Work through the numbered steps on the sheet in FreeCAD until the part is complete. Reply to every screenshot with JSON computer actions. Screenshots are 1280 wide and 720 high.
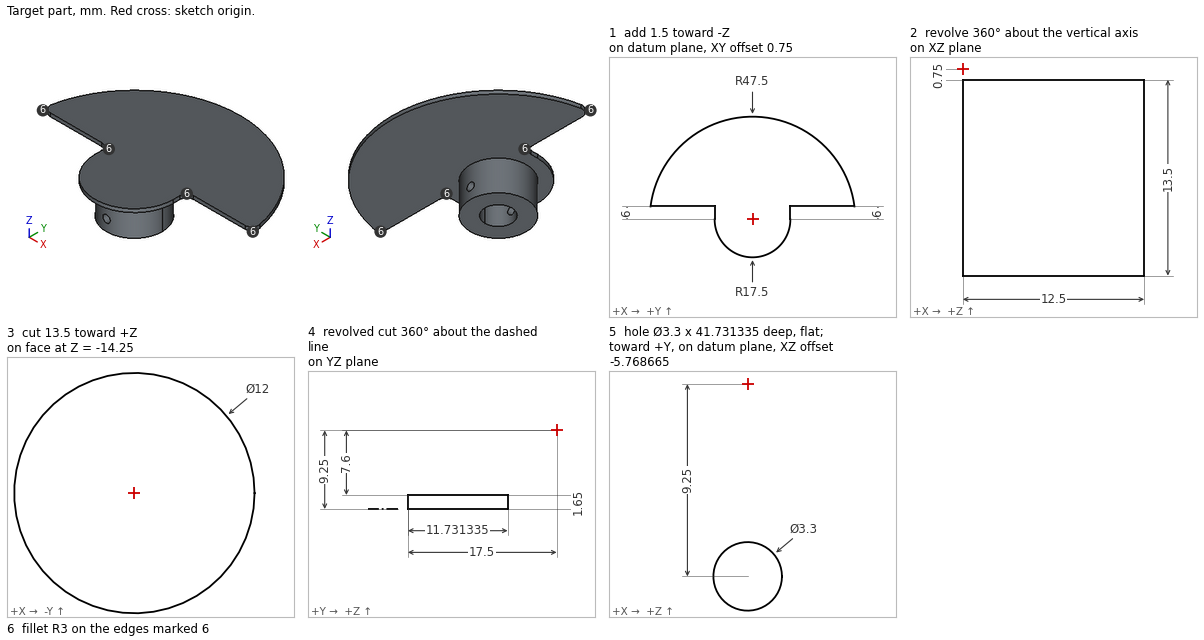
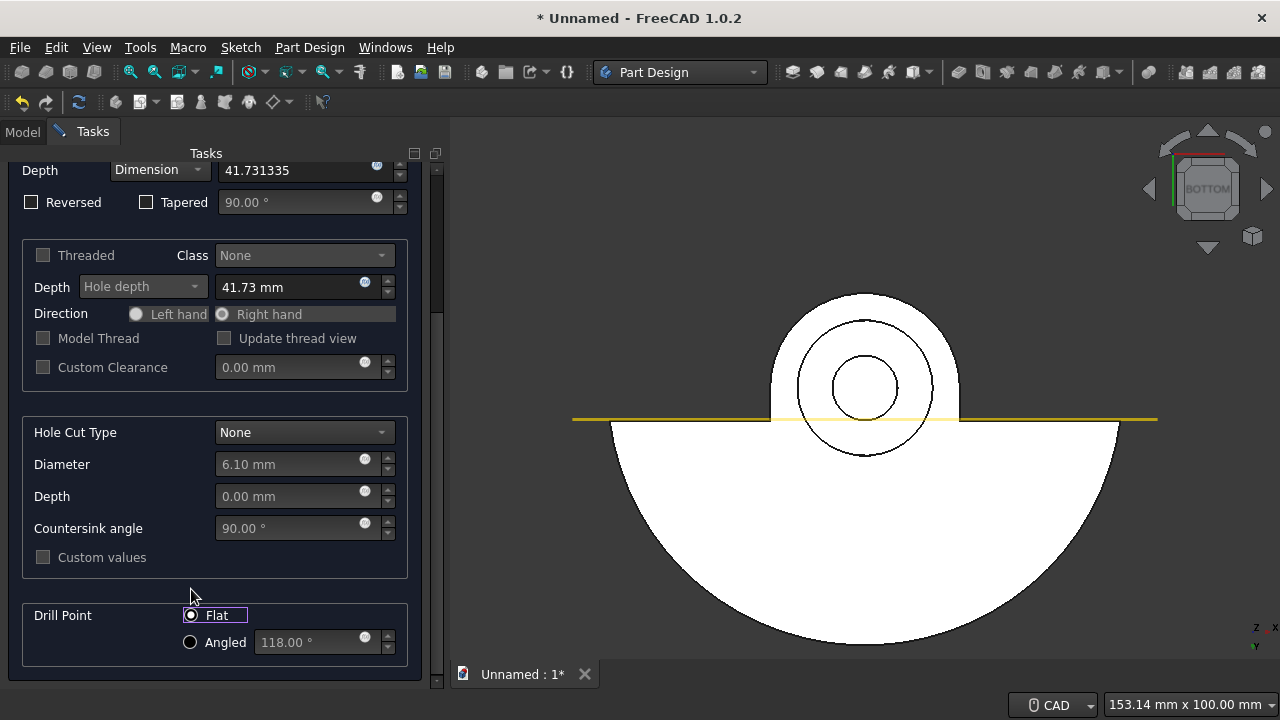
{"action": "scroll", "coordinate": [437, 426], "scroll_direction": "up", "scroll_amount": 5}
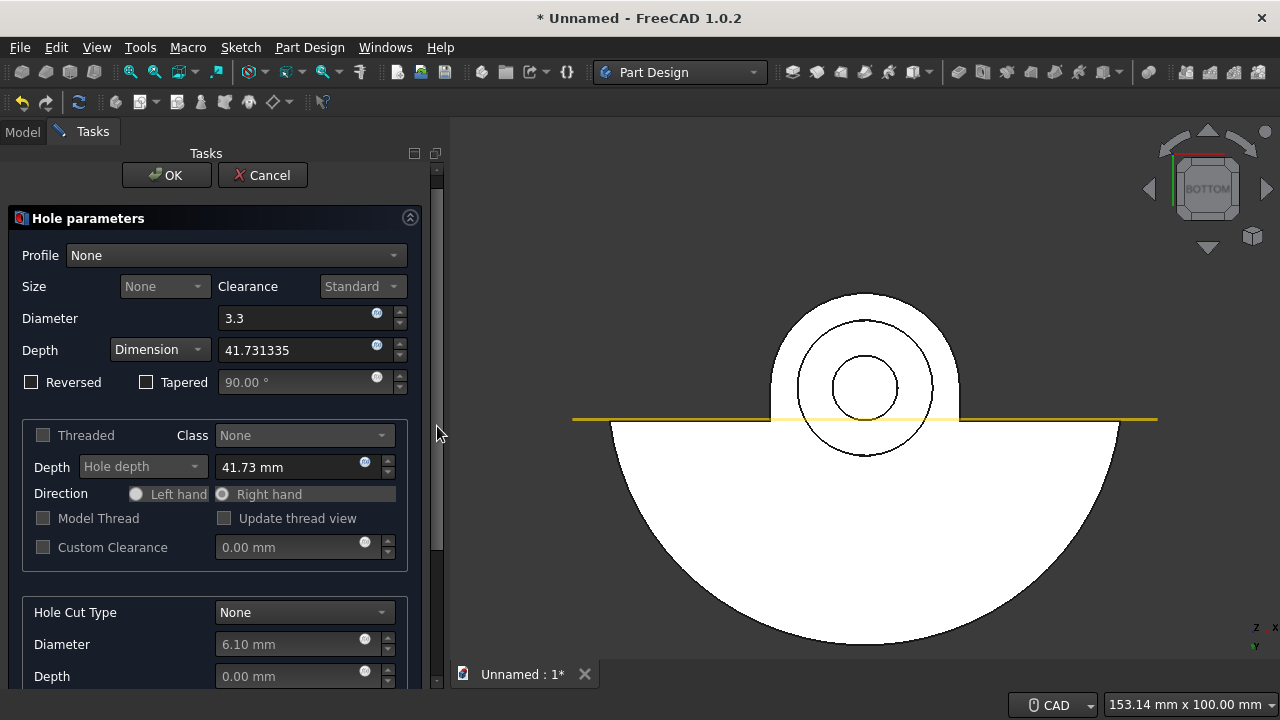
{"action": "left_click", "coordinate": [167, 192]}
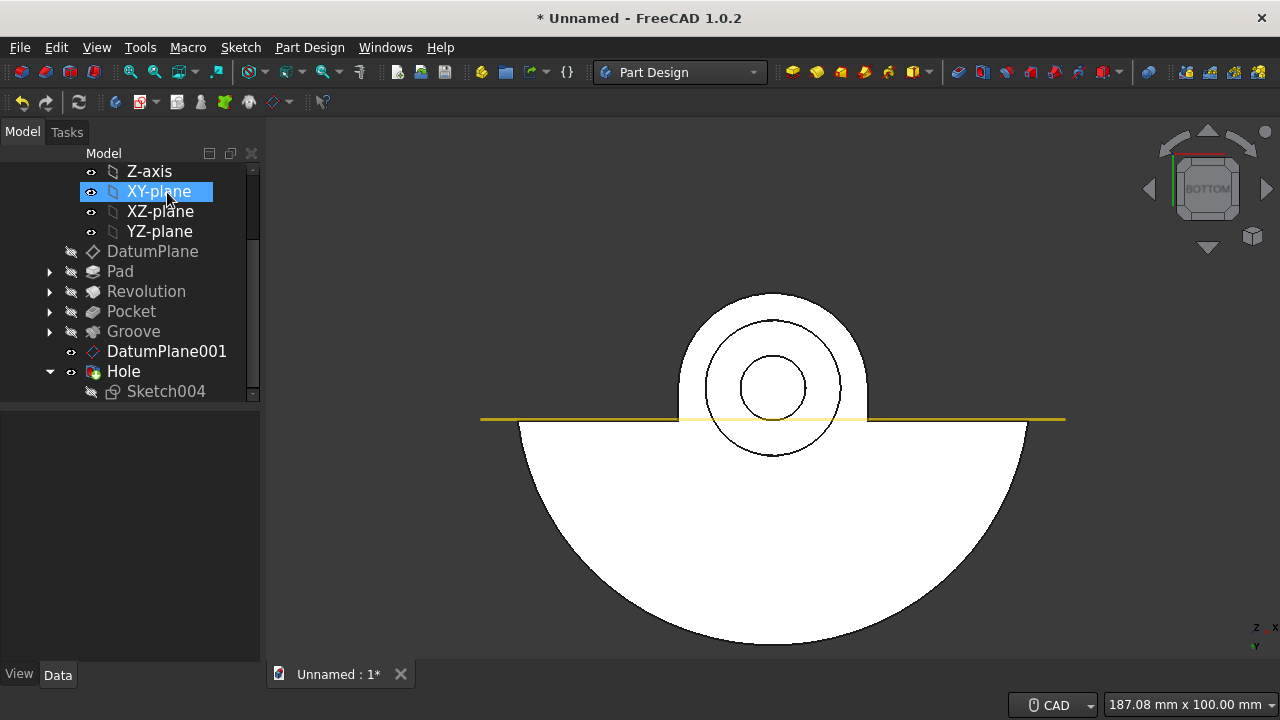
{"action": "left_click", "coordinate": [116, 352]}
{"action": "key", "text": "space"}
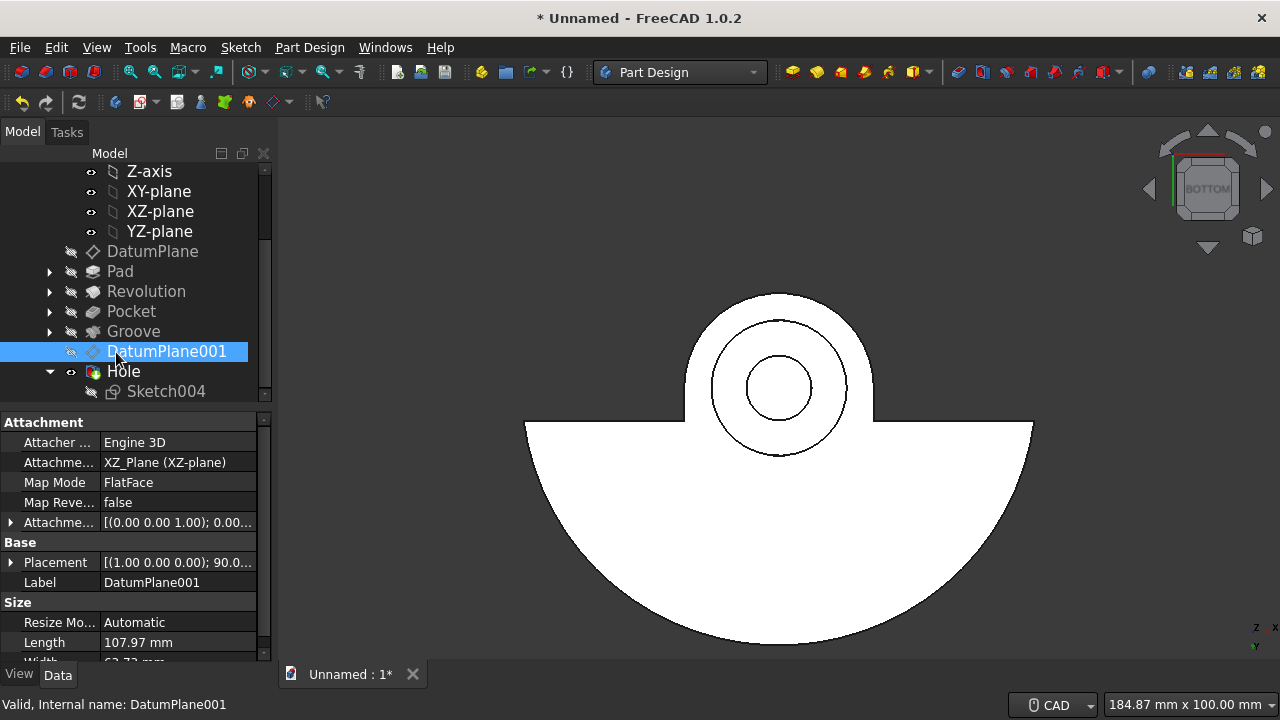
{"action": "scroll", "coordinate": [684, 420], "scroll_direction": "up", "scroll_amount": 8}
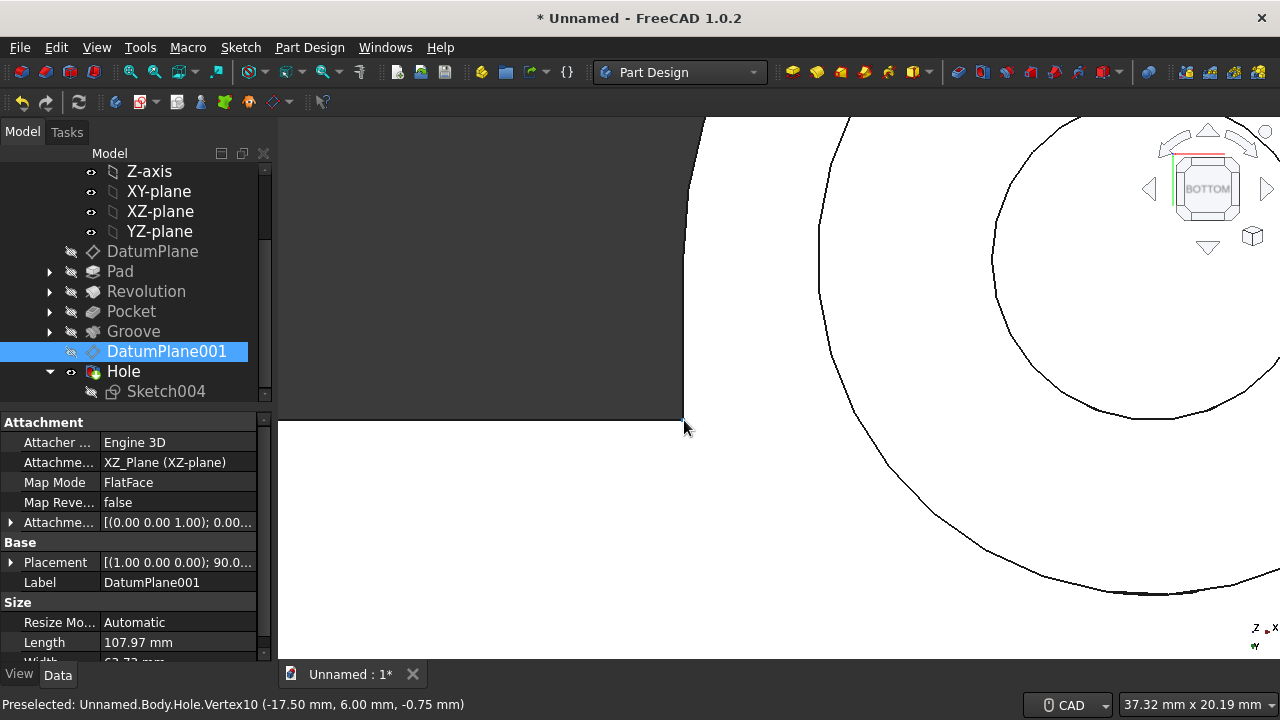
{"action": "key", "text": "v f"}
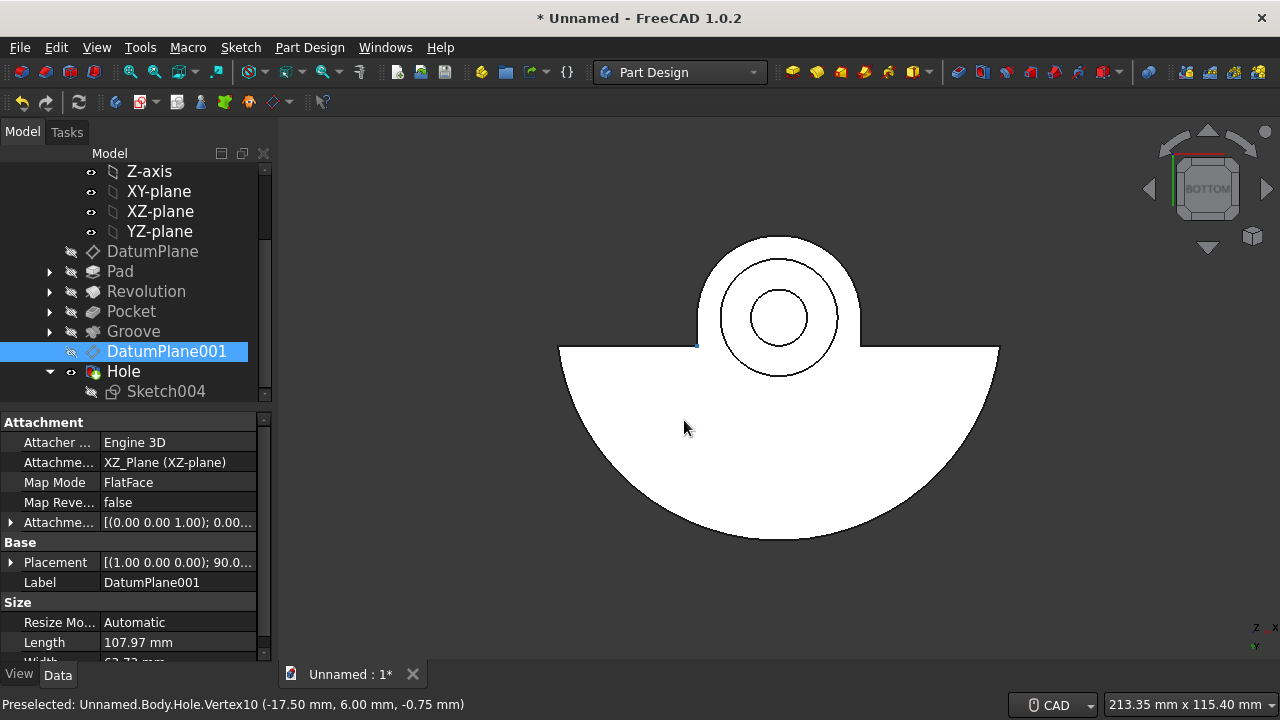
{"action": "key", "text": "0"}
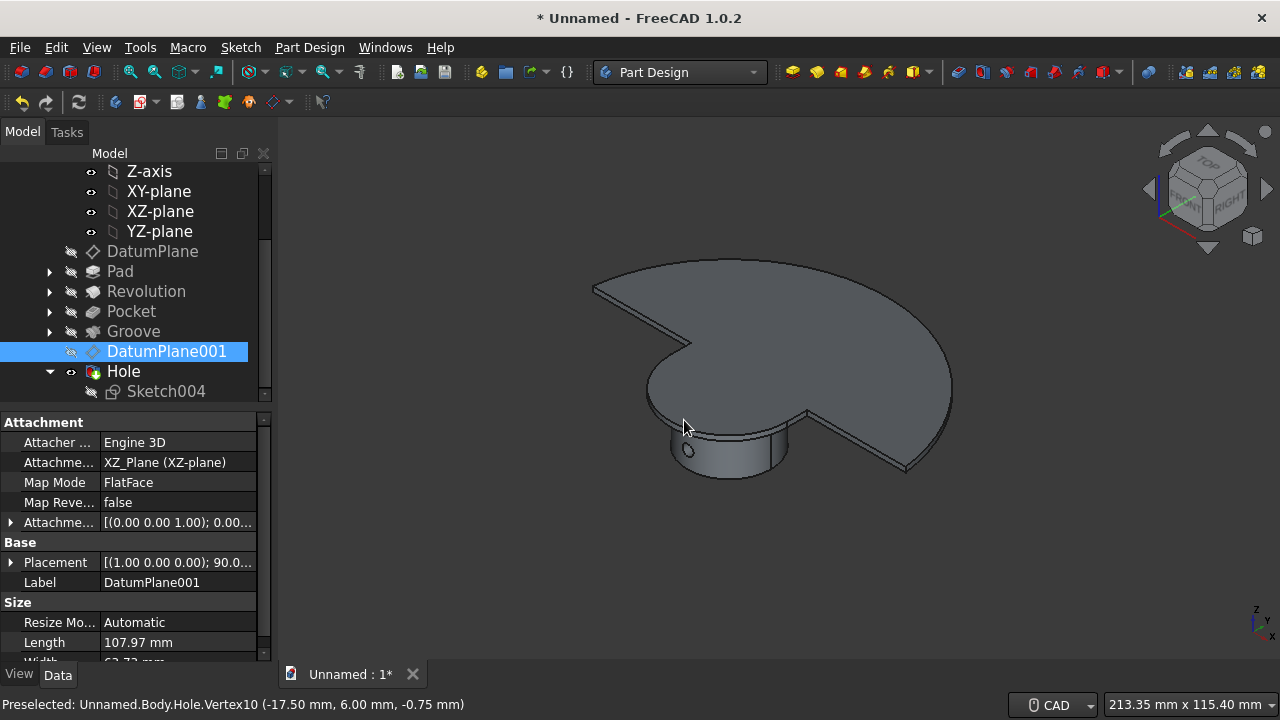
{"action": "scroll", "coordinate": [691, 345], "scroll_direction": "up", "scroll_amount": 9}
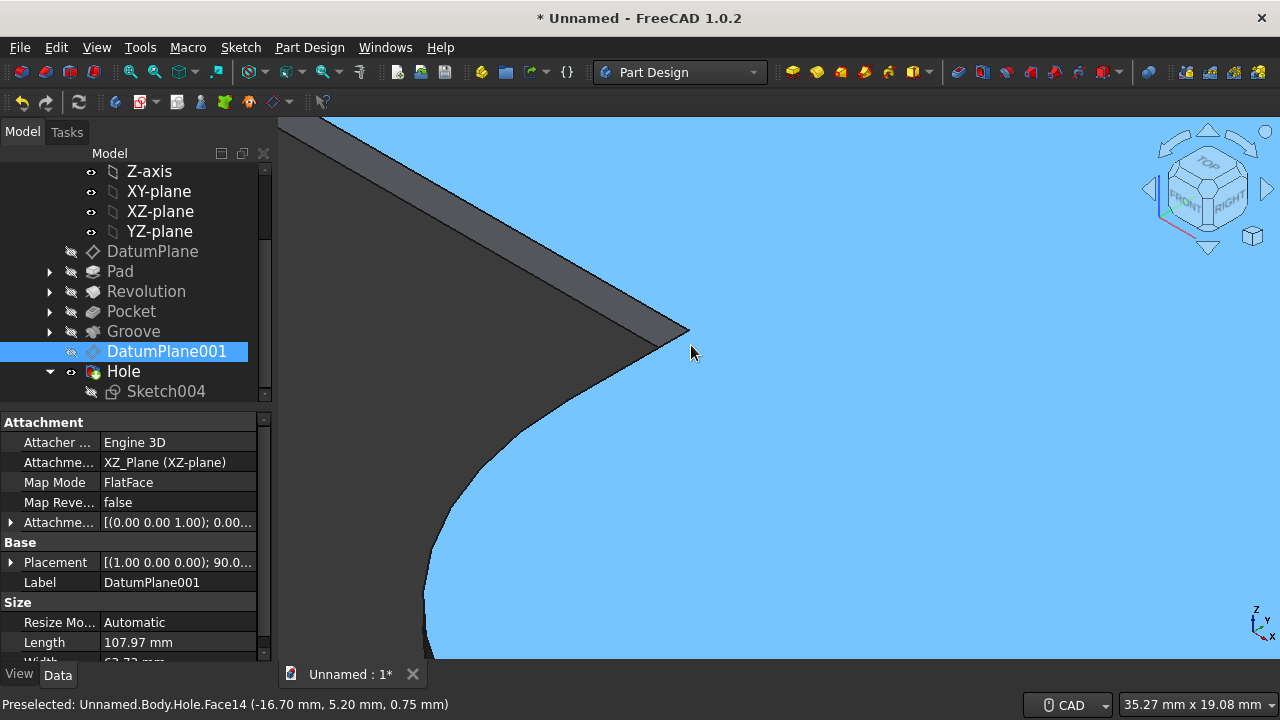
{"action": "left_click", "coordinate": [132, 72]}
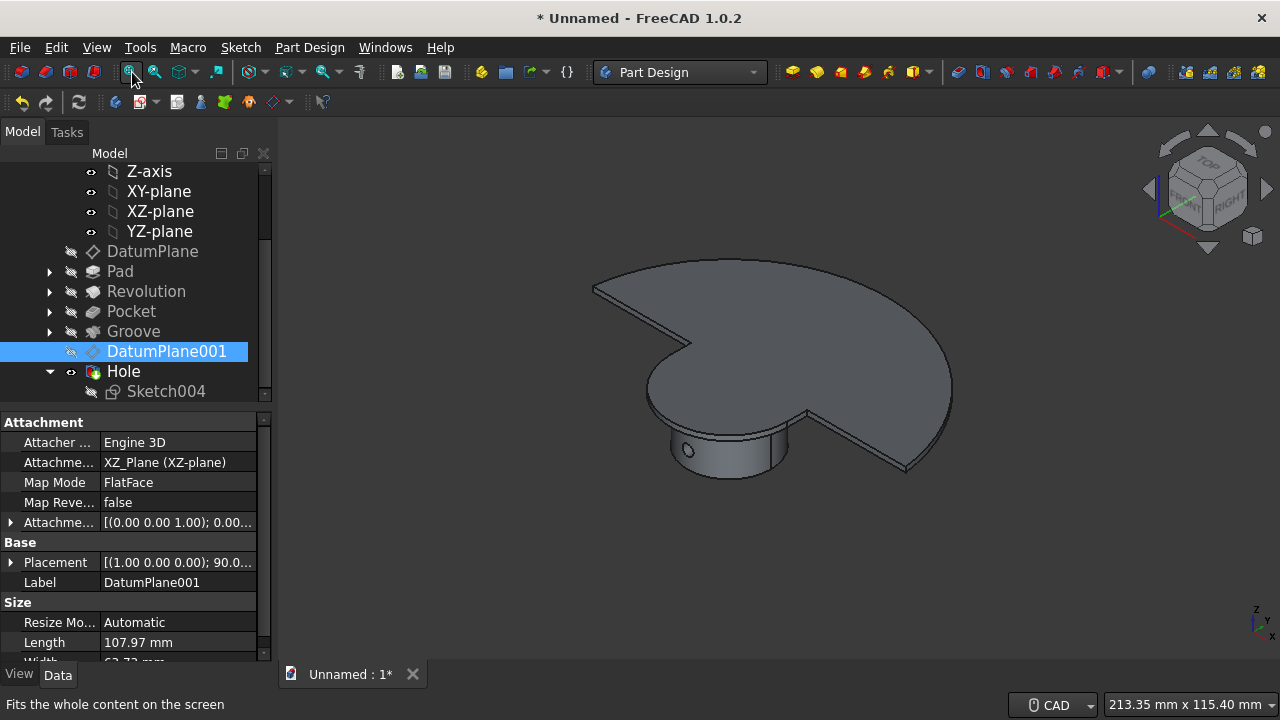
{"action": "key", "text": "2"}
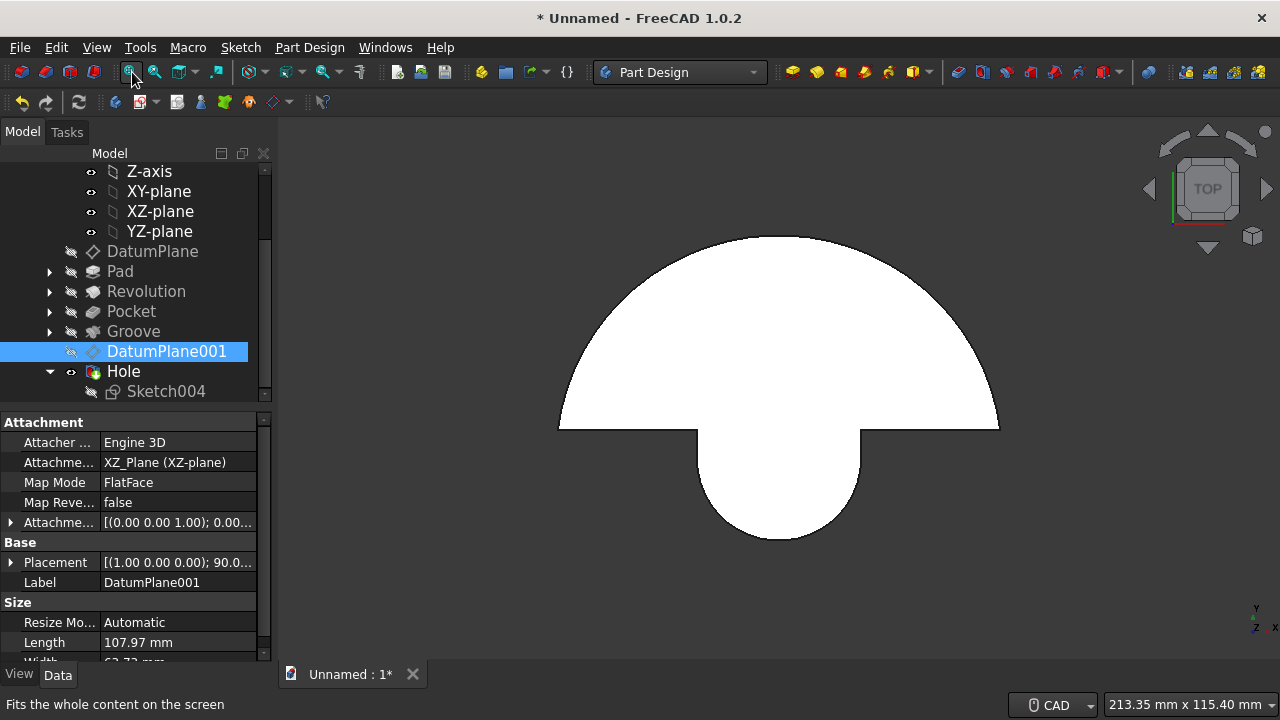
{"action": "scroll", "coordinate": [697, 429], "scroll_direction": "up", "scroll_amount": 9}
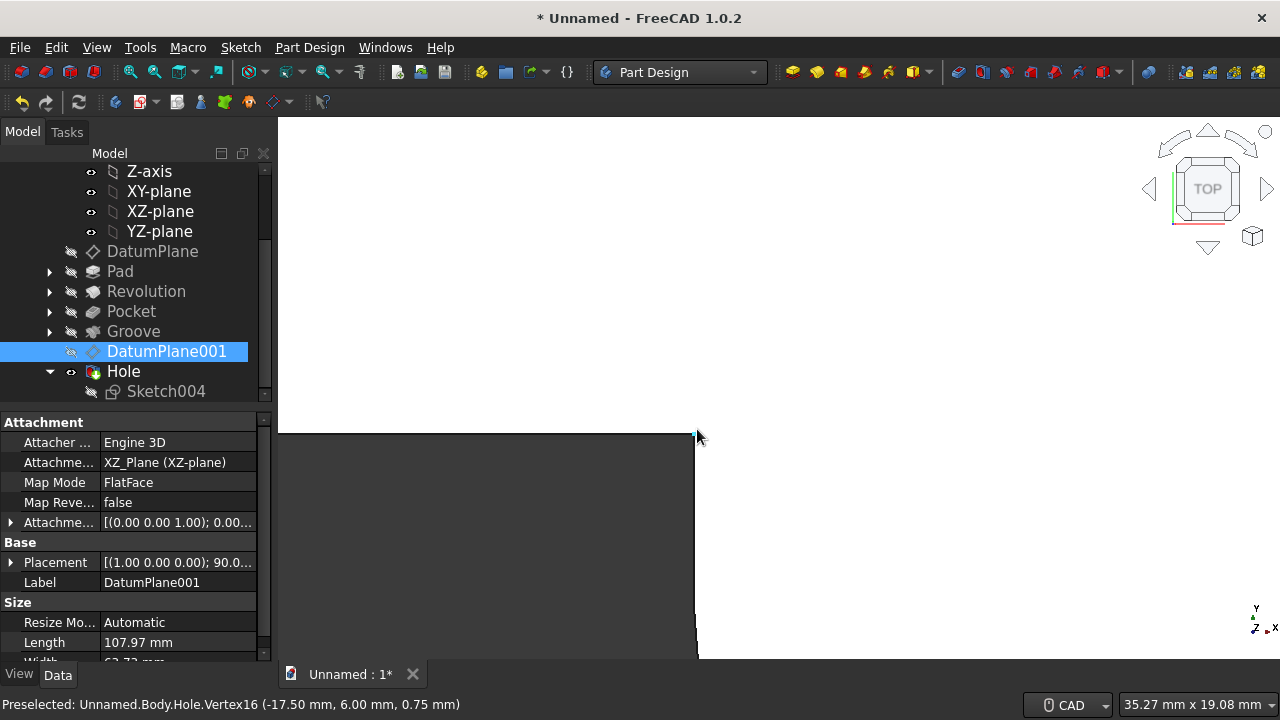
{"action": "key", "text": "v f"}